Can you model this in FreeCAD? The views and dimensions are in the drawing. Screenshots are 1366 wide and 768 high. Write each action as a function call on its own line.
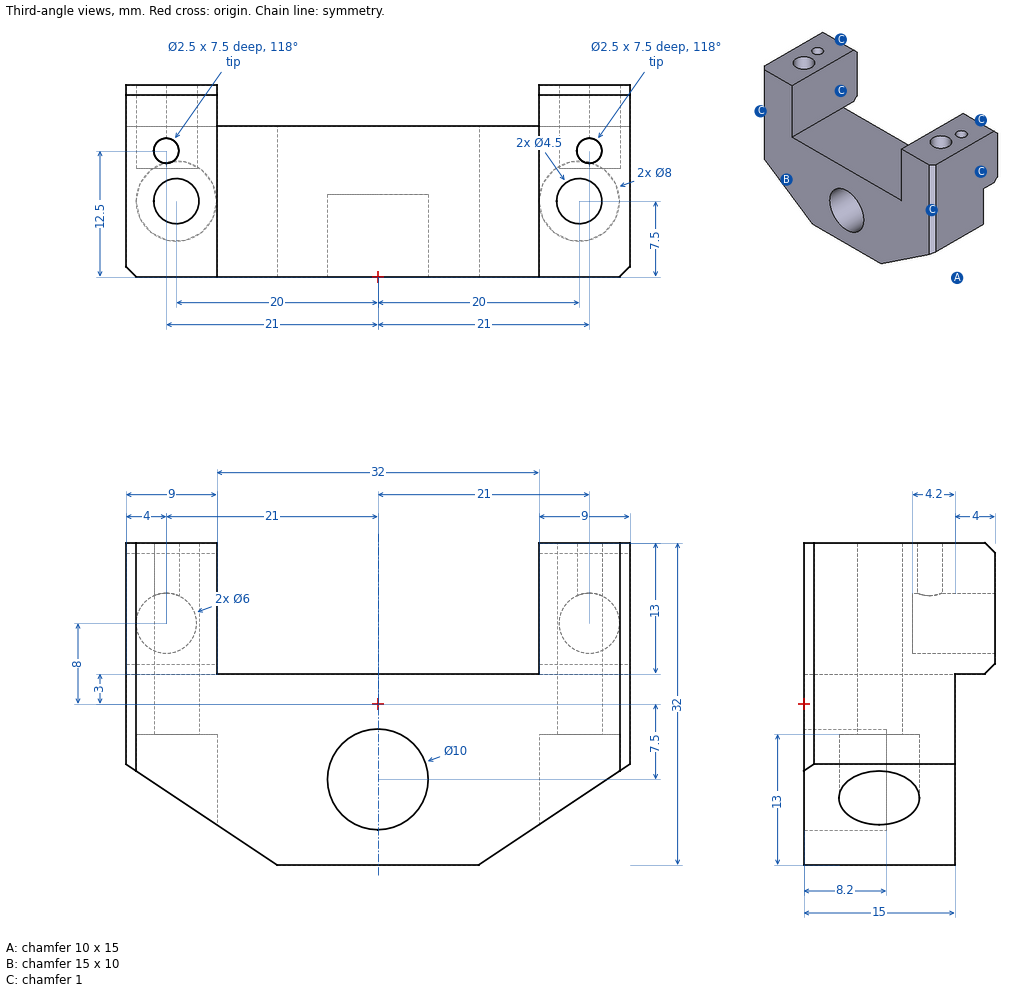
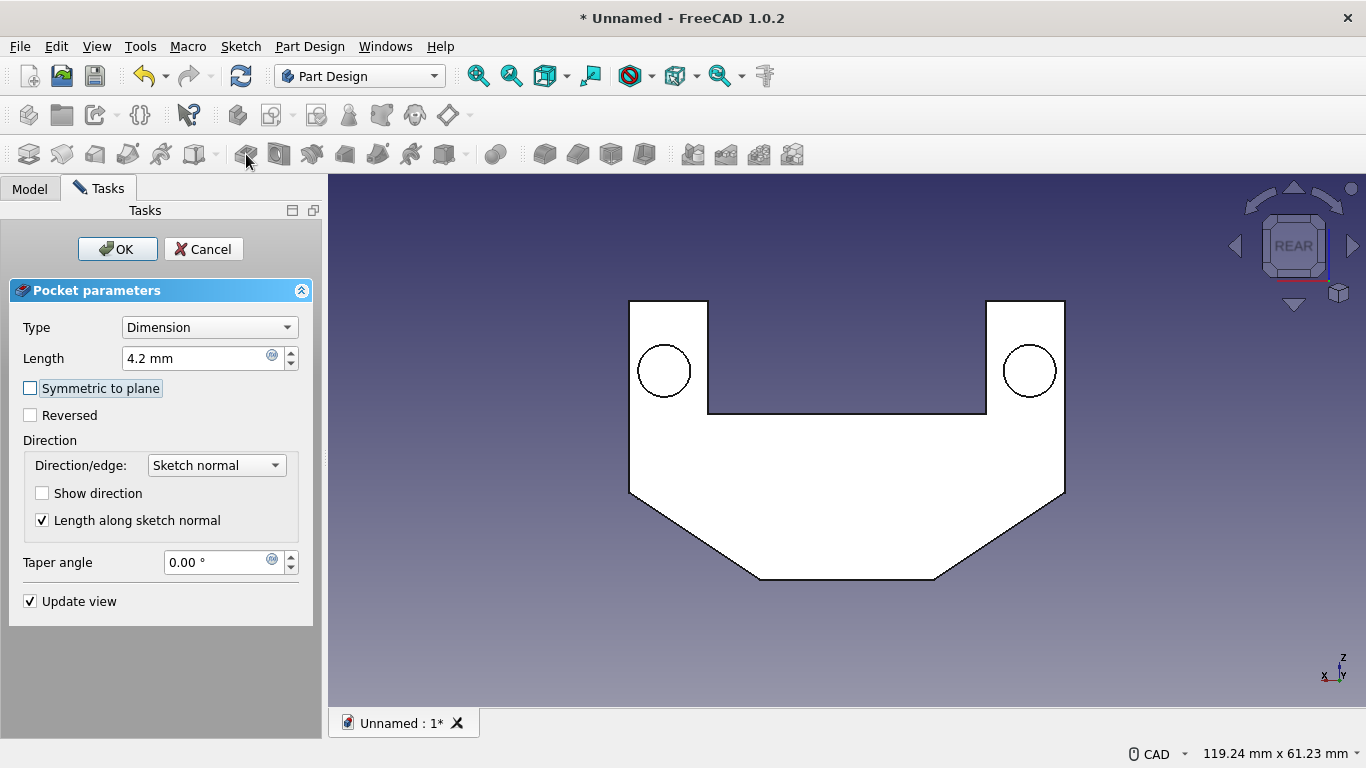
click(118, 249)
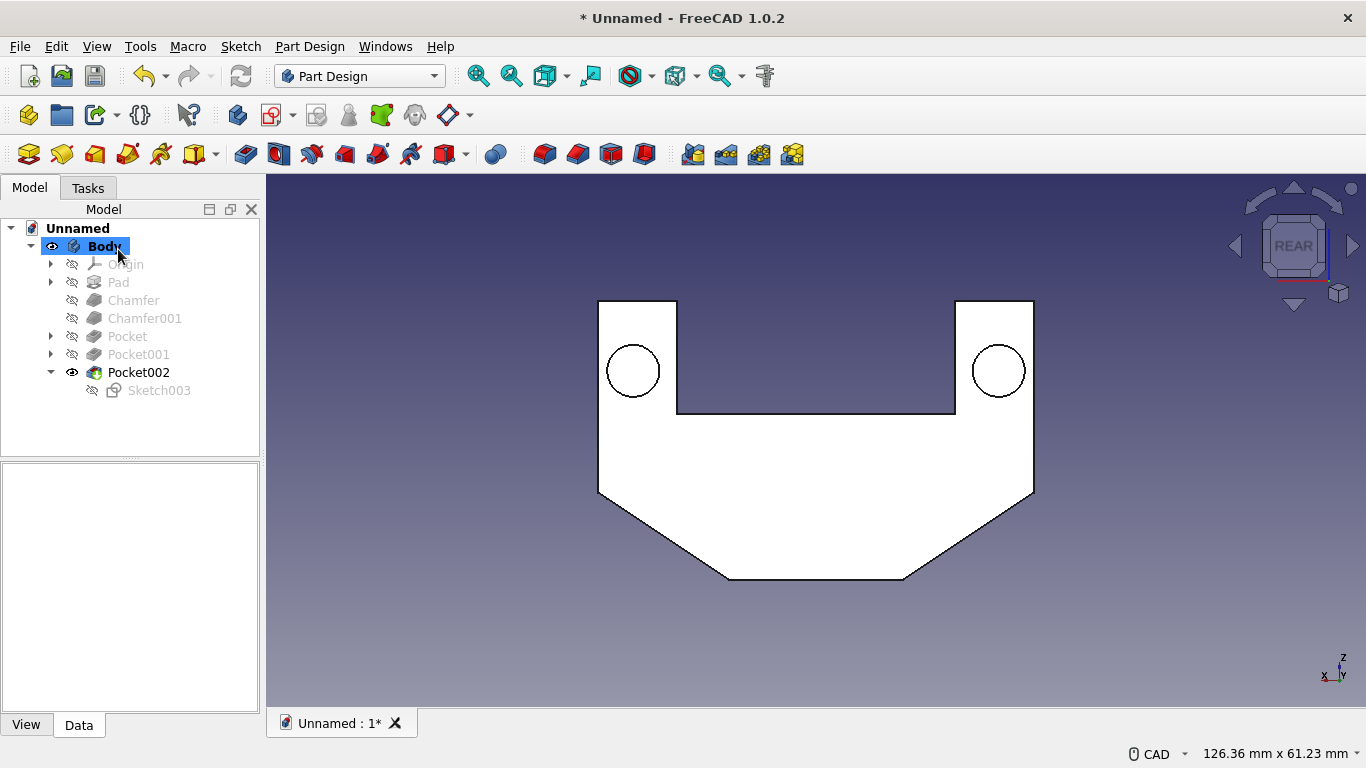
key(0)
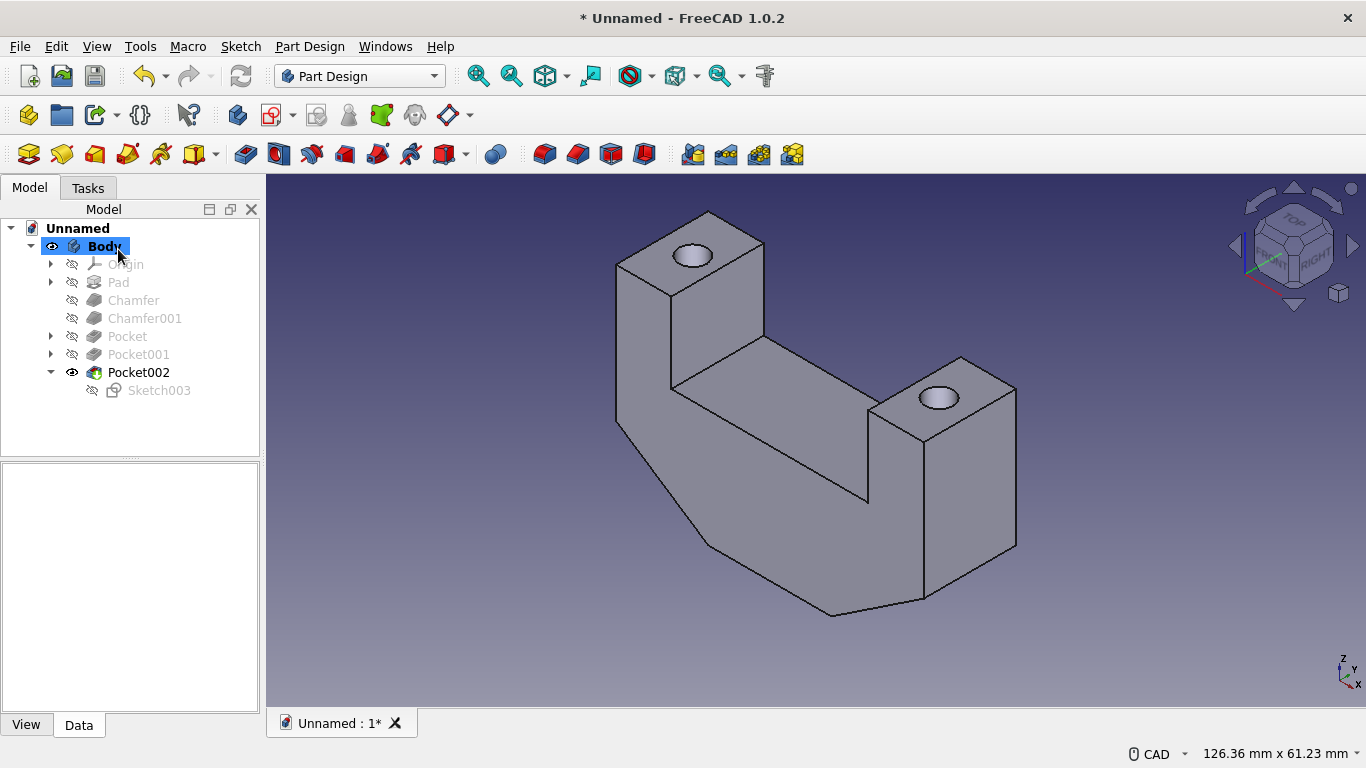
click(976, 388)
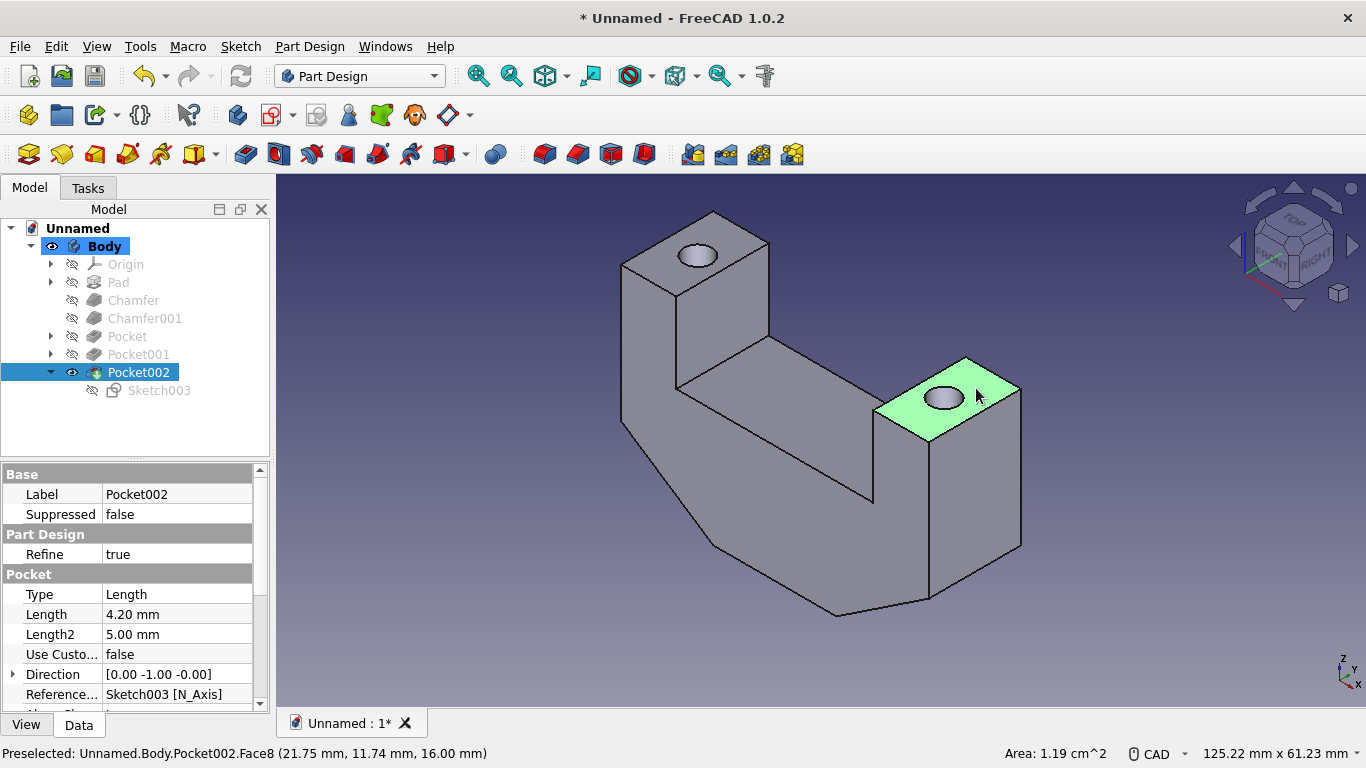
click(270, 116)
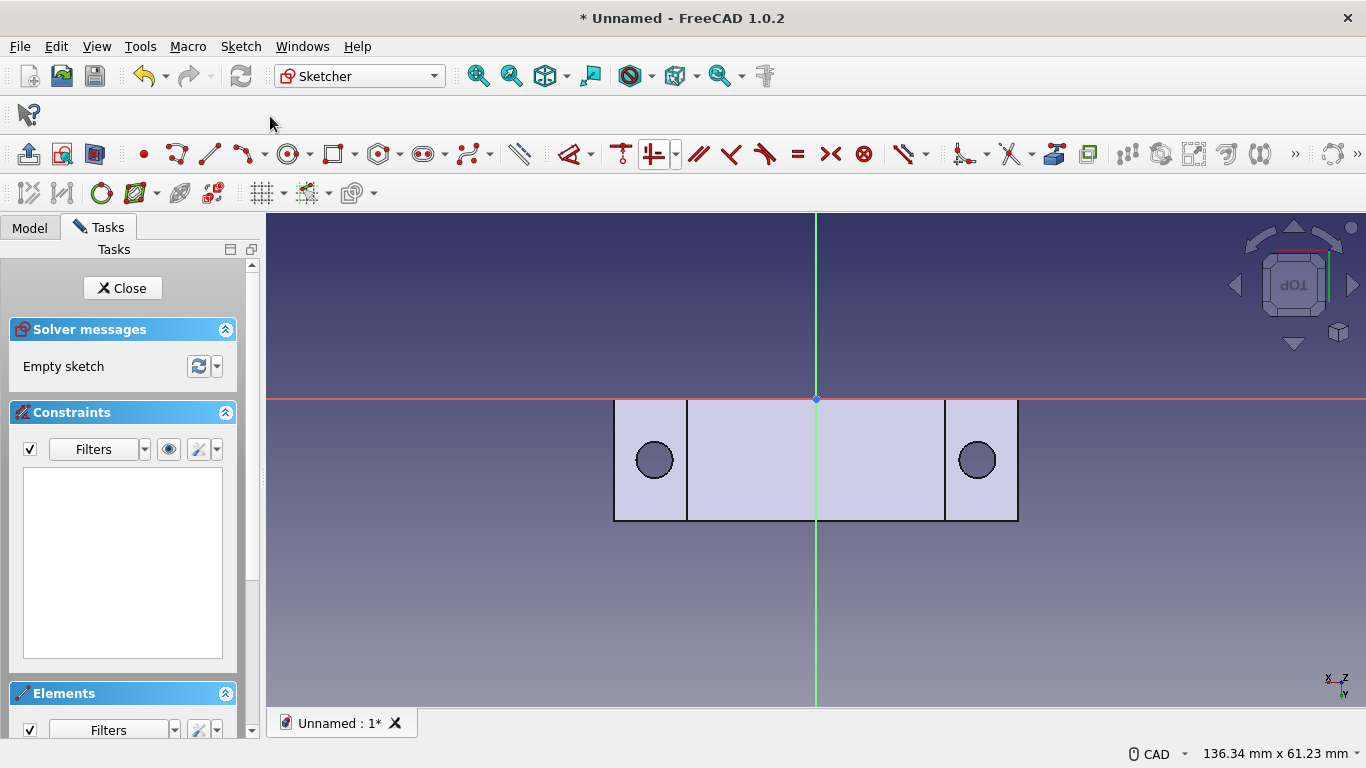
scroll(1001, 503, up, 14)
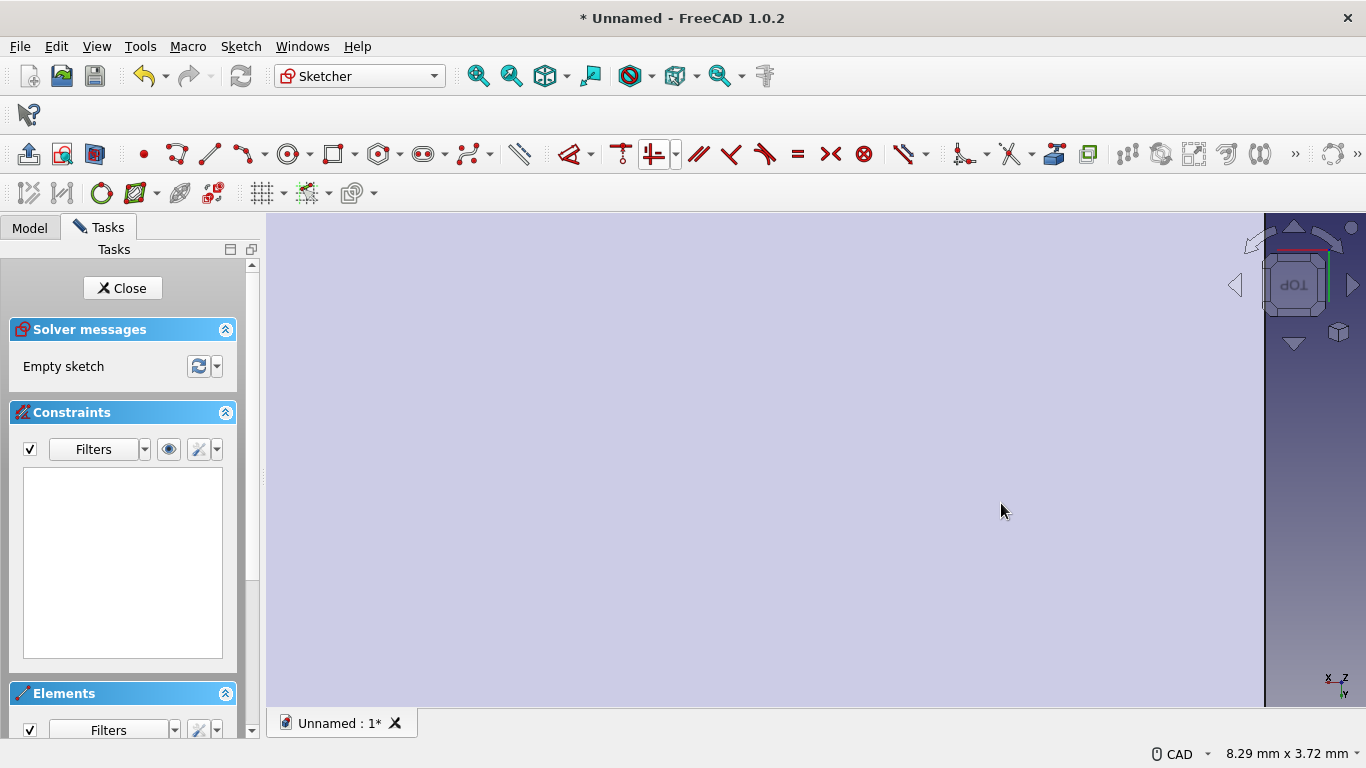
click(288, 154)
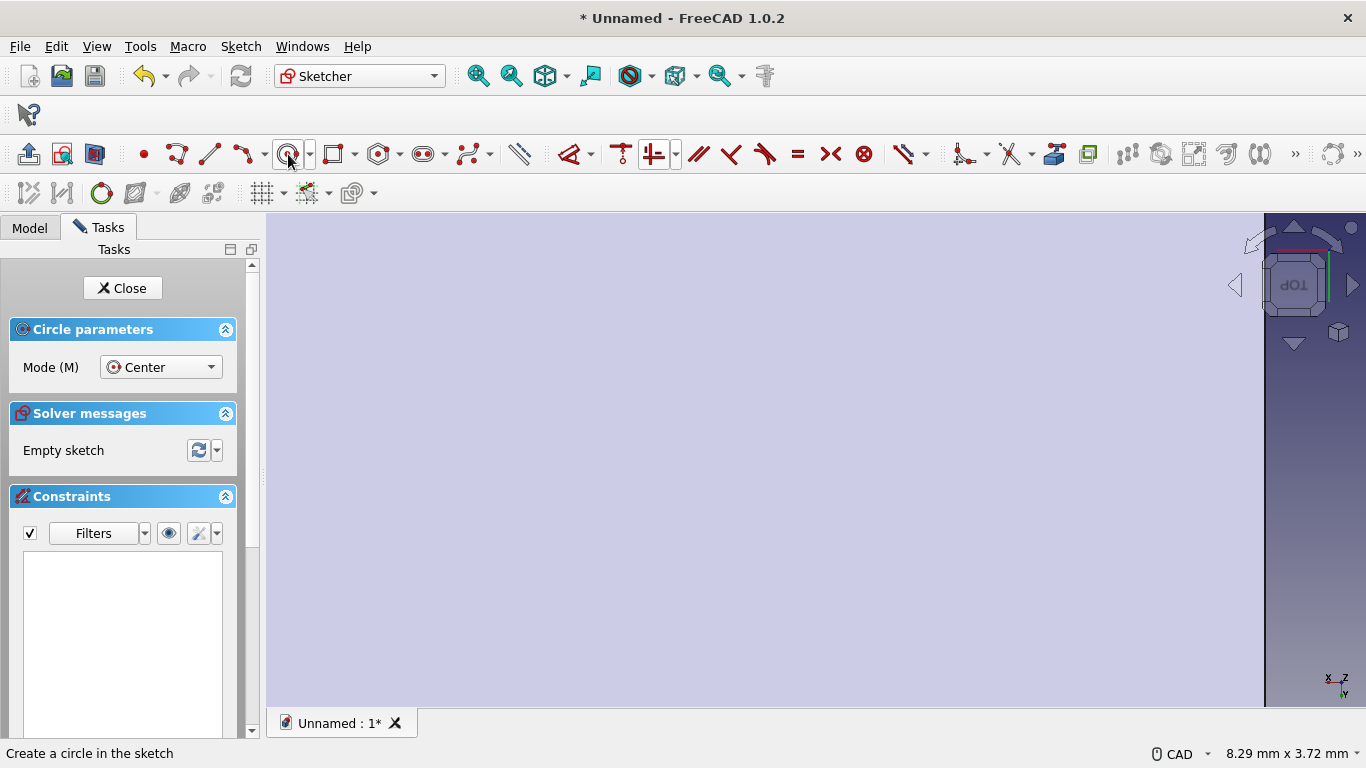
click(735, 450)
move(852, 333)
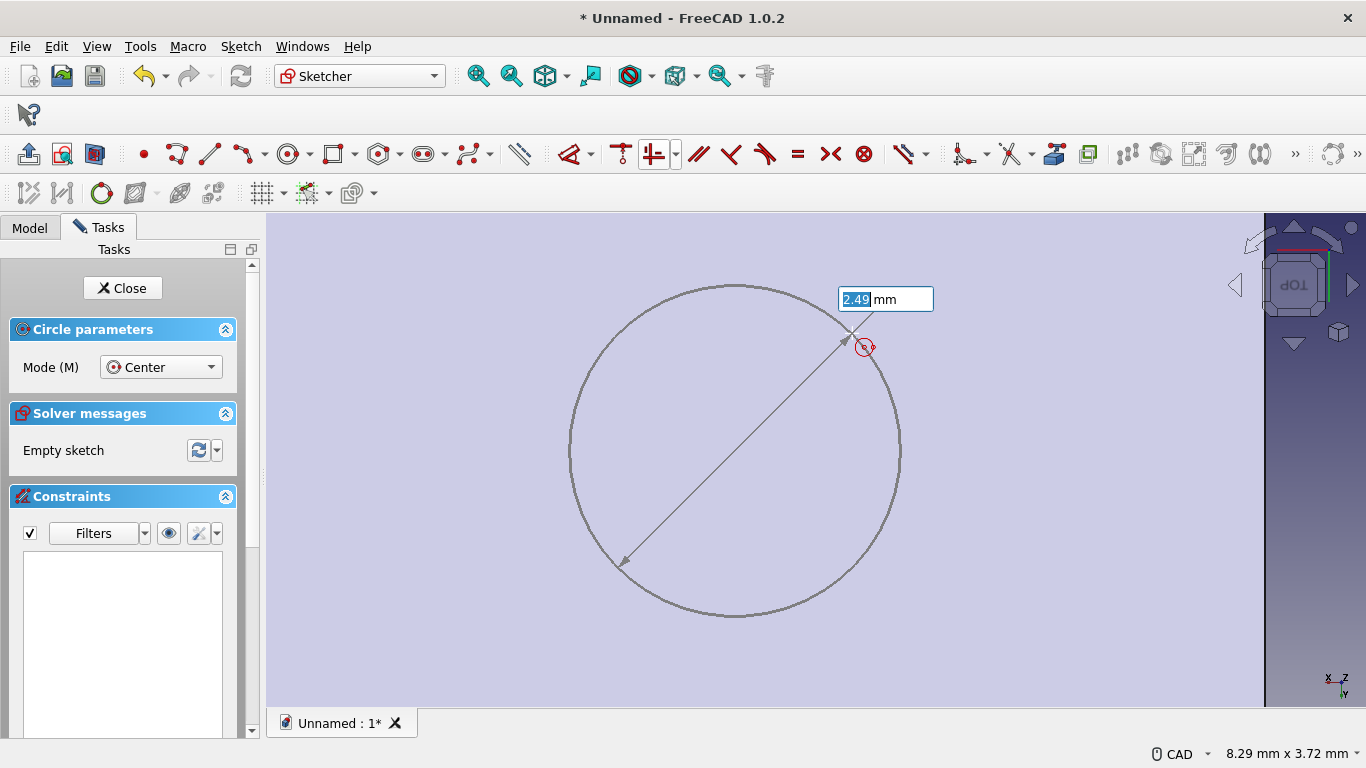
text(2.5)
key(Return)
key(Escape)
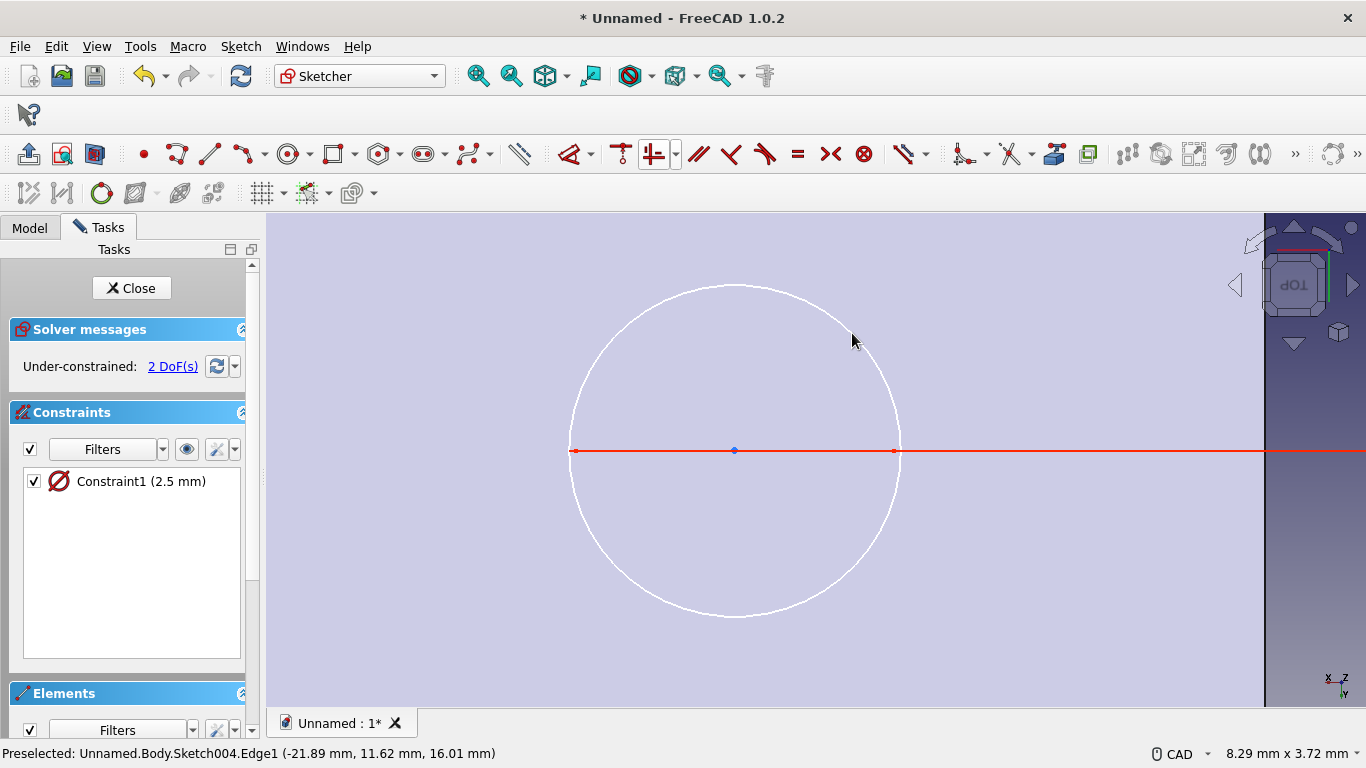
click(568, 154)